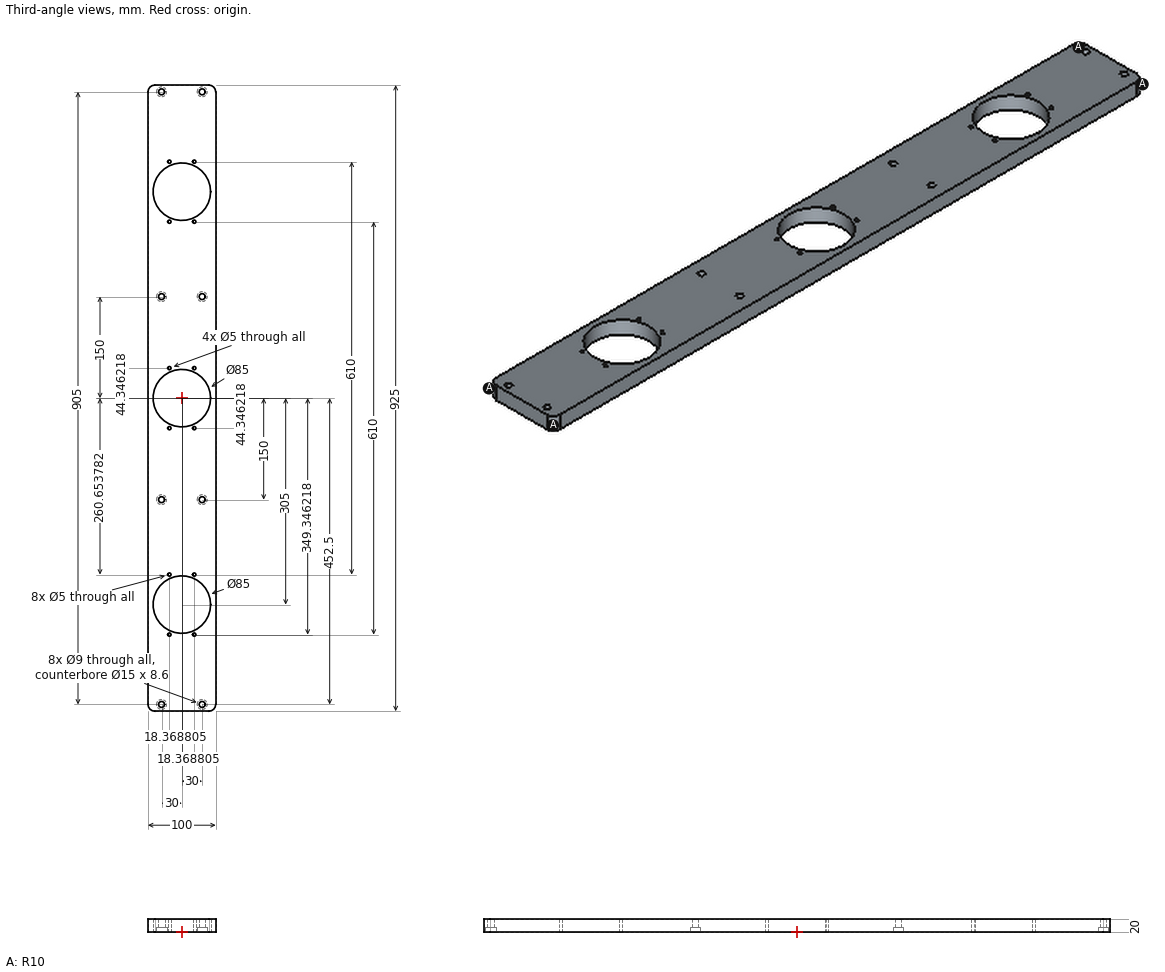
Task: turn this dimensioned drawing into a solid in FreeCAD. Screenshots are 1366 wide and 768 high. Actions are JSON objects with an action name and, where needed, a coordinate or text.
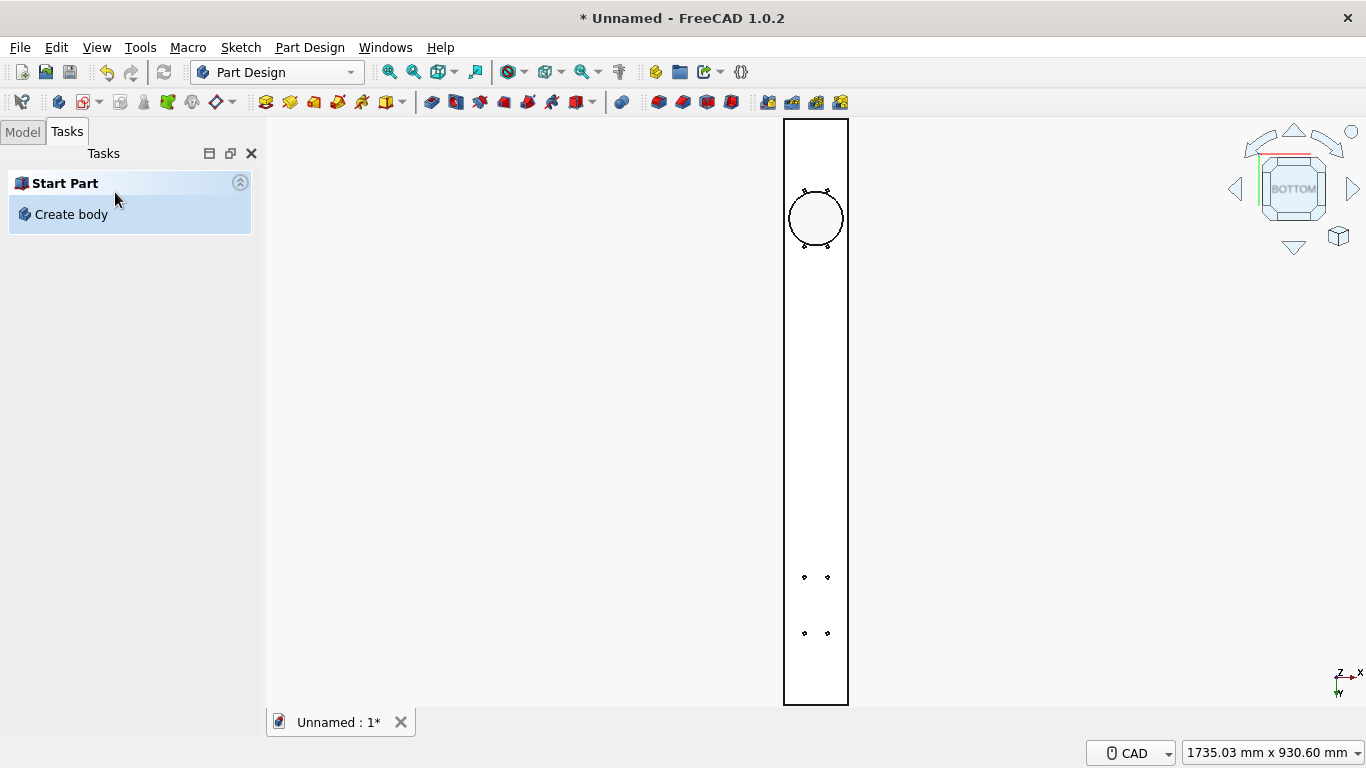
{"action": "left_click", "coordinate": [816, 495]}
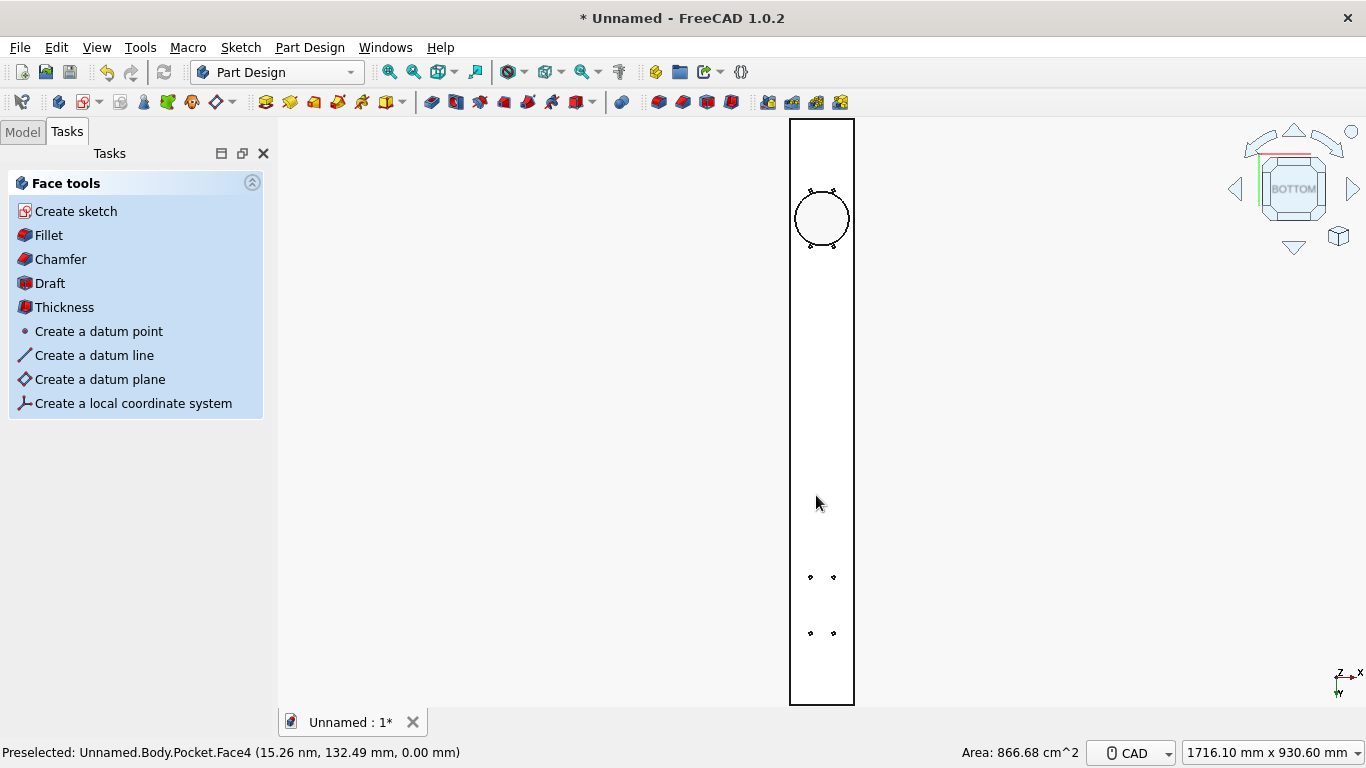
{"action": "left_click", "coordinate": [84, 102]}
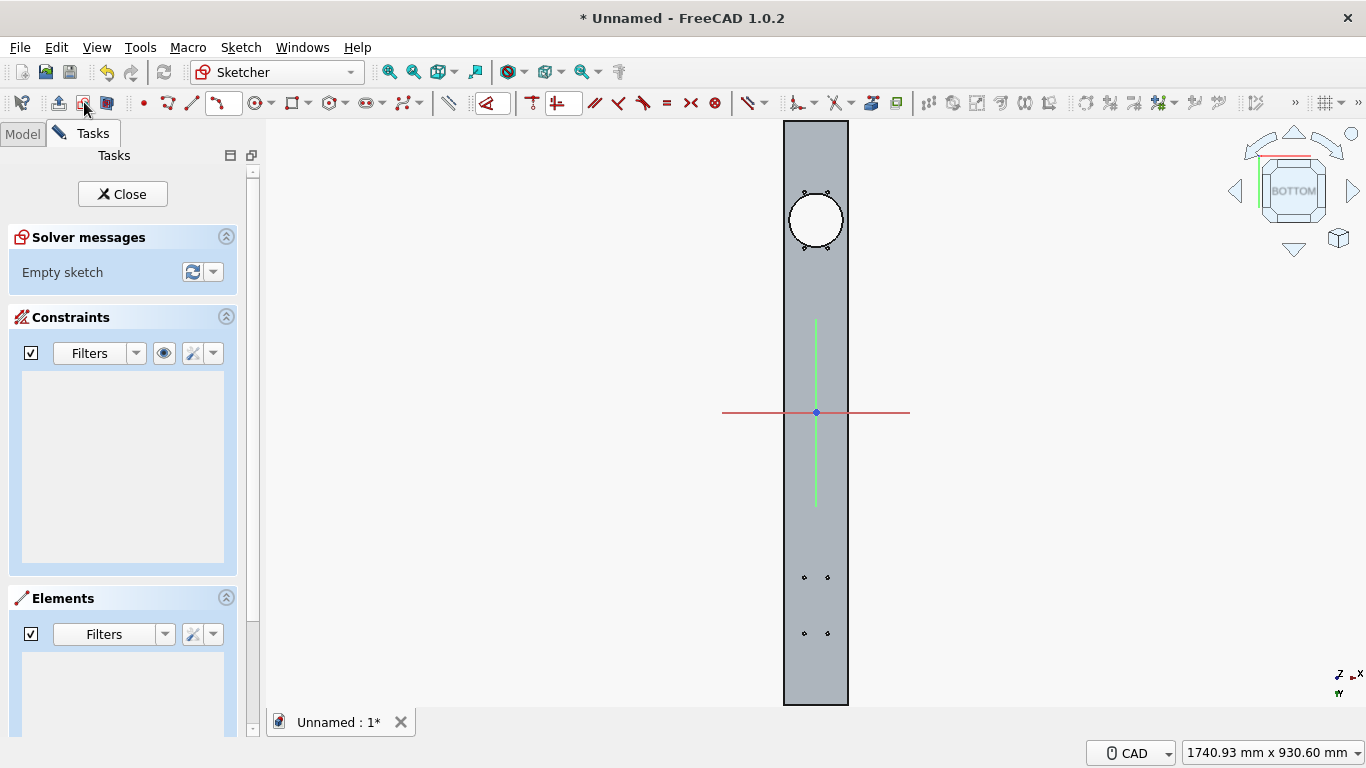
{"action": "scroll", "coordinate": [608, 413], "scroll_direction": "down", "scroll_amount": 2}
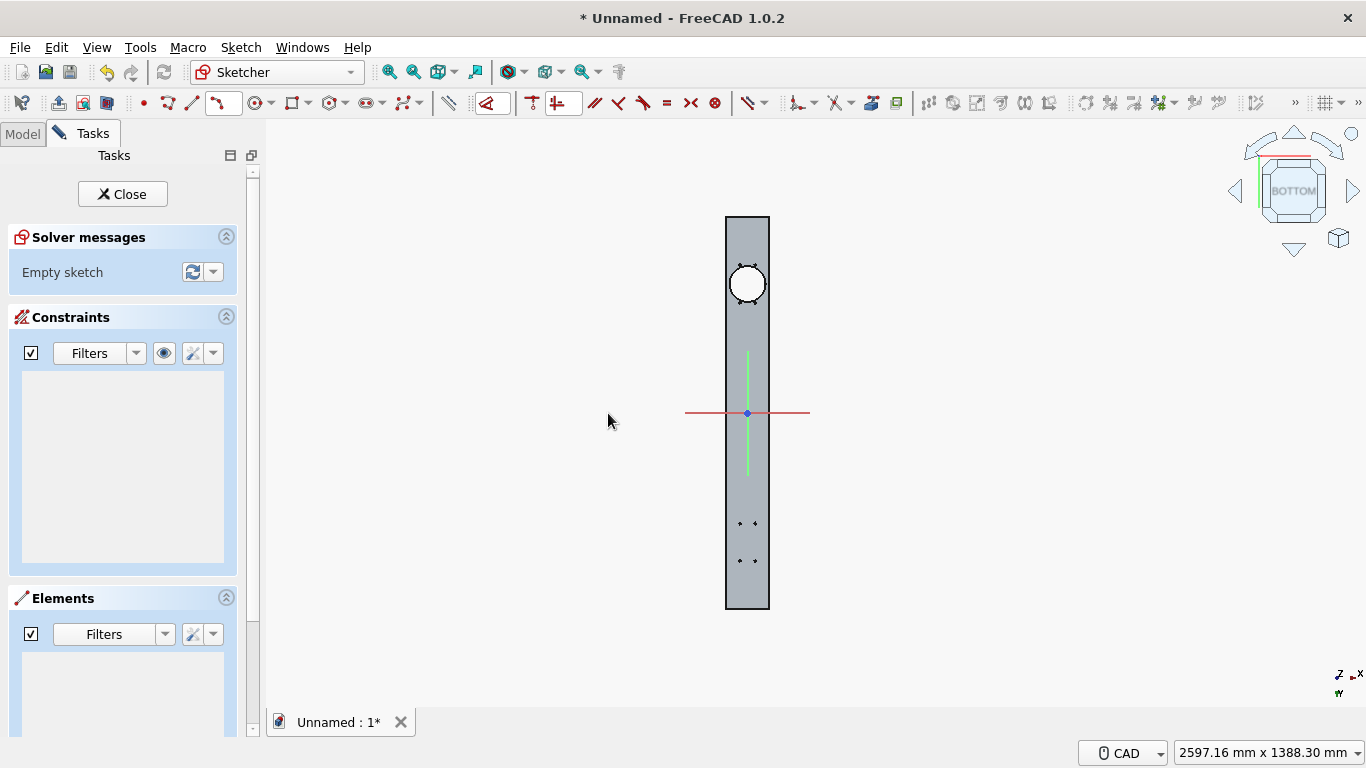
{"action": "key", "text": "g c"}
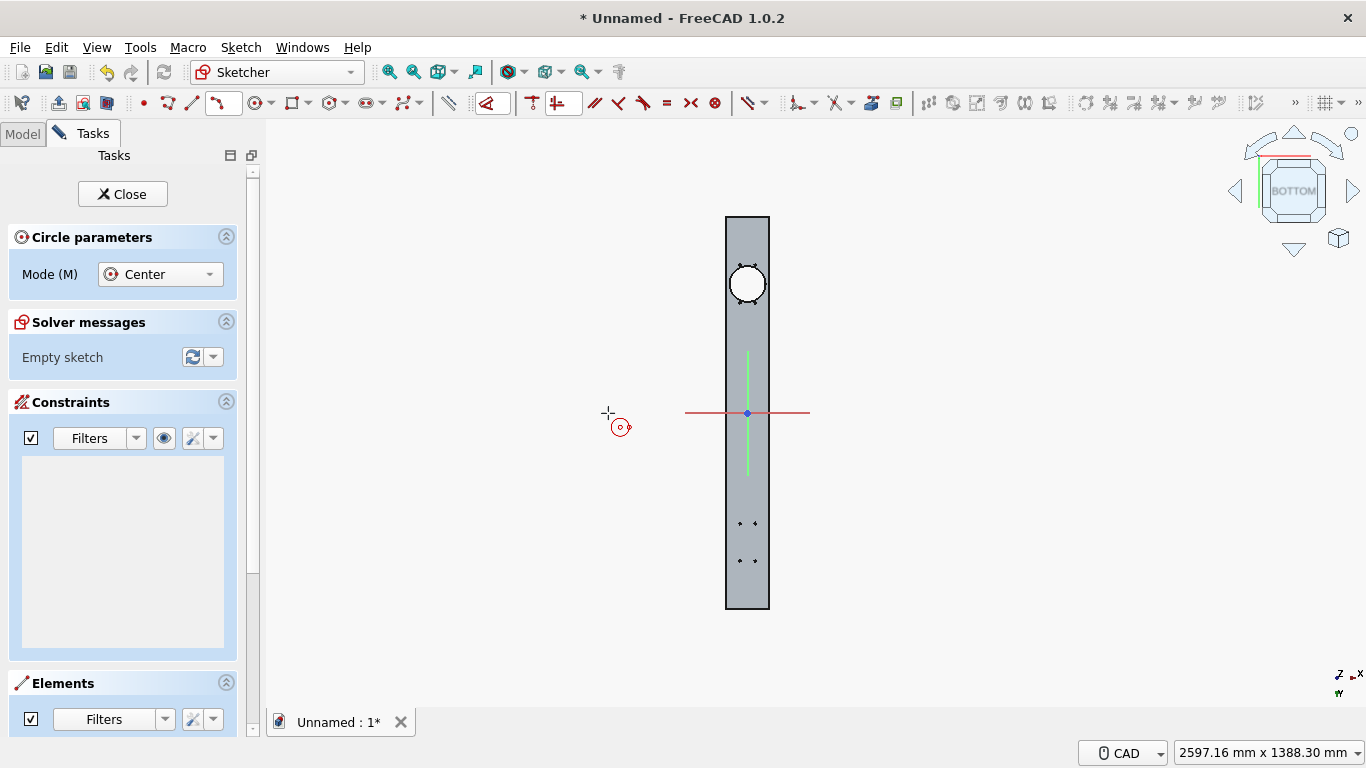
{"action": "scroll", "coordinate": [760, 222], "scroll_direction": "up", "scroll_amount": 13}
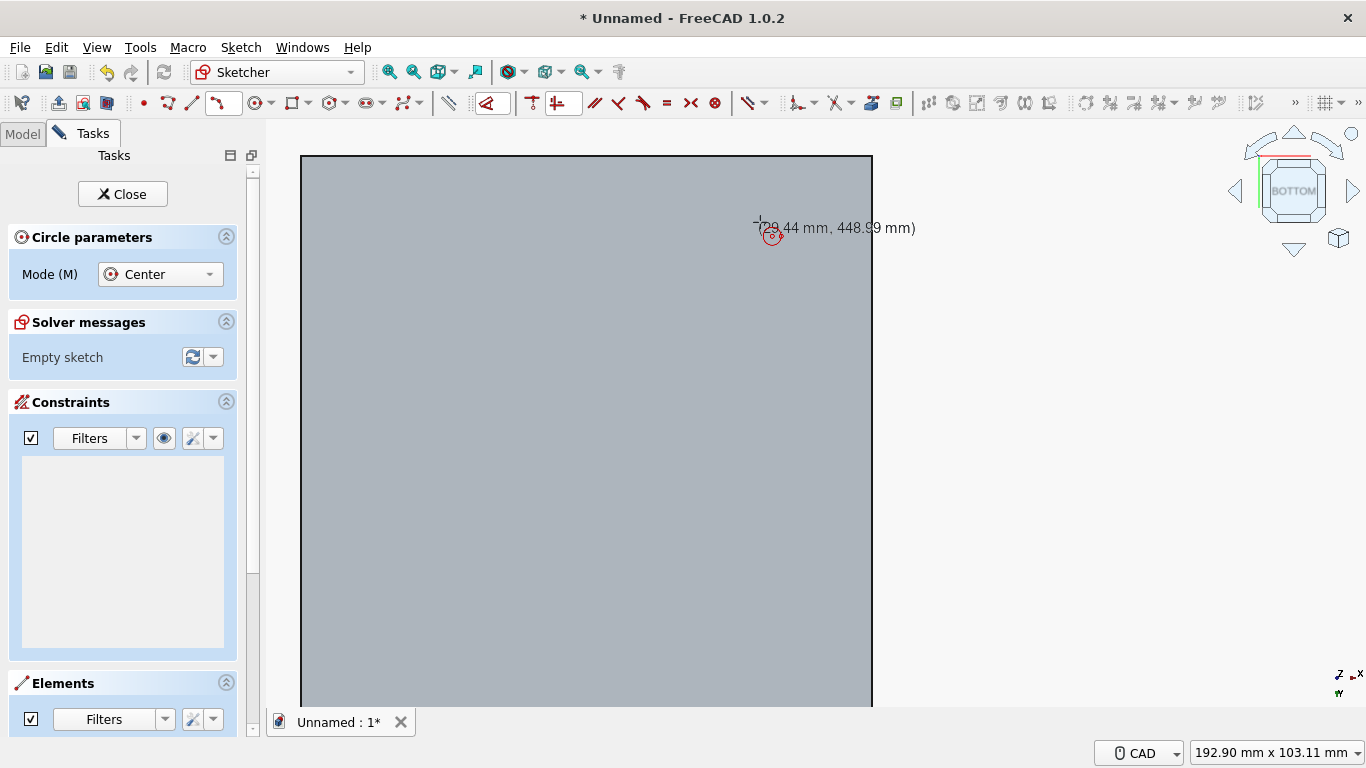
{"action": "scroll", "coordinate": [760, 222], "scroll_direction": "down", "scroll_amount": 13}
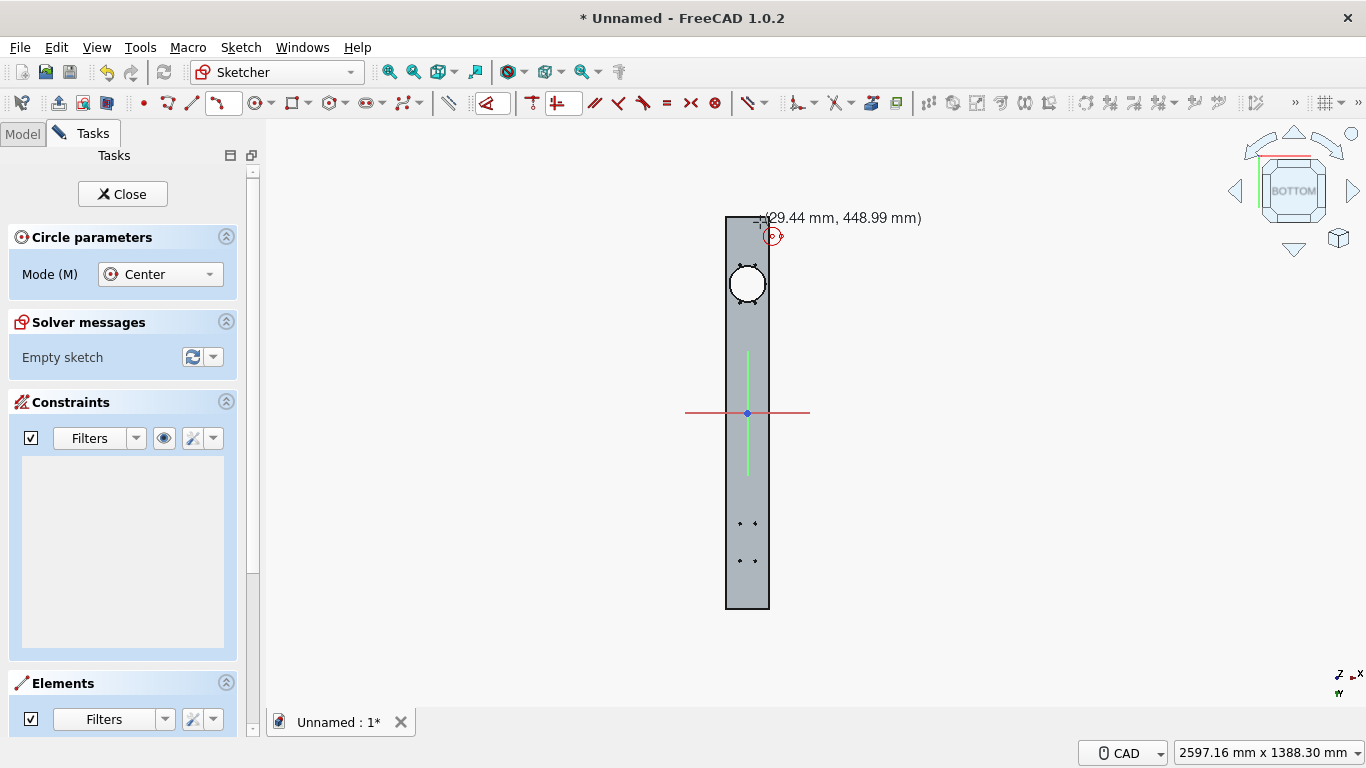
{"action": "scroll", "coordinate": [760, 222], "scroll_direction": "up", "scroll_amount": 2}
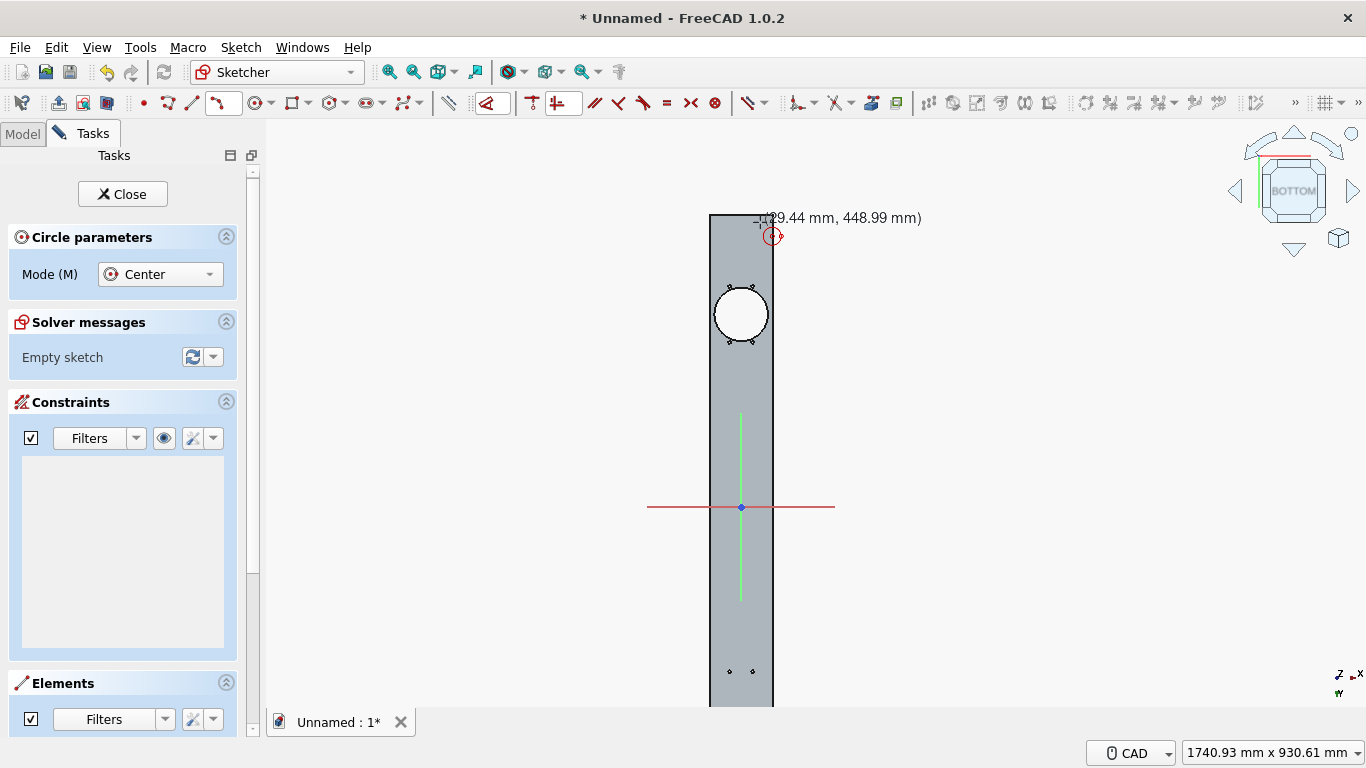
{"action": "left_click", "coordinate": [760, 221]}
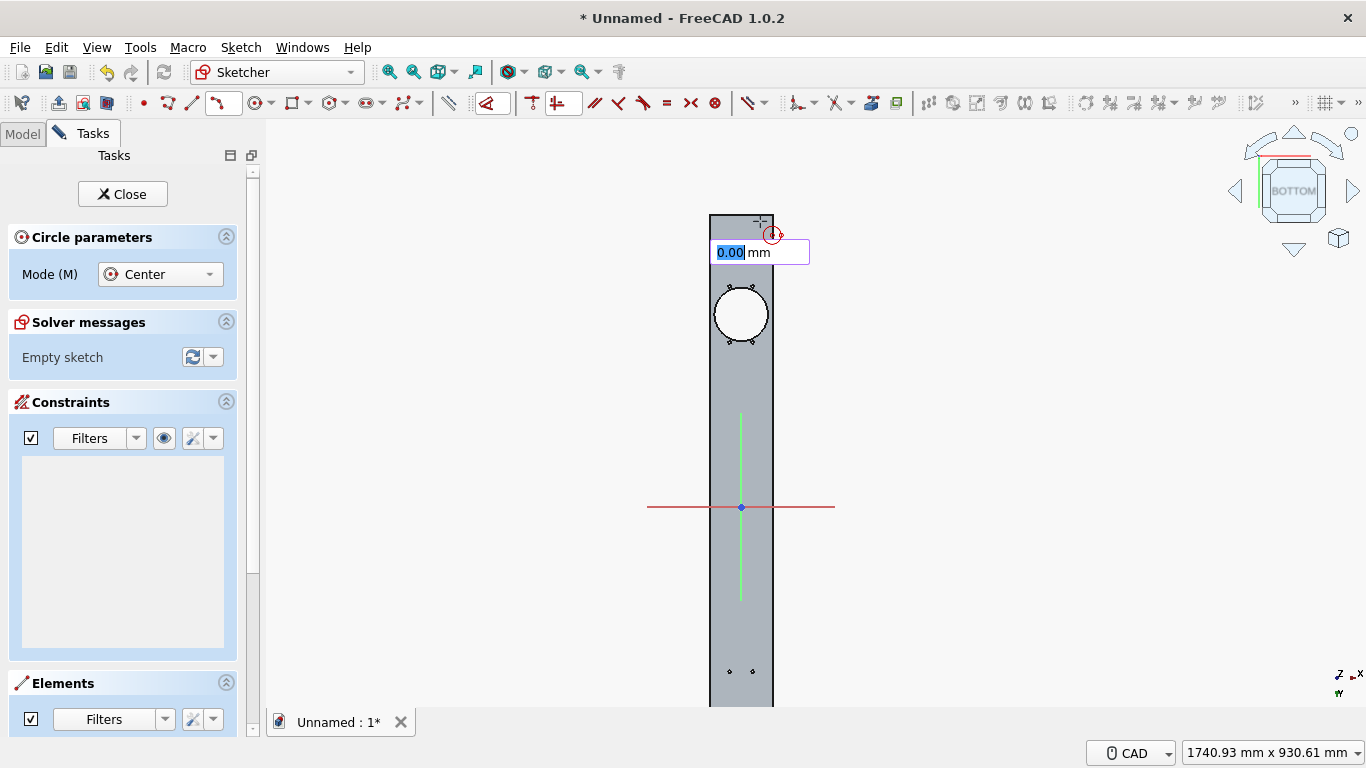
{"action": "scroll", "coordinate": [762, 219], "scroll_direction": "up", "scroll_amount": 9}